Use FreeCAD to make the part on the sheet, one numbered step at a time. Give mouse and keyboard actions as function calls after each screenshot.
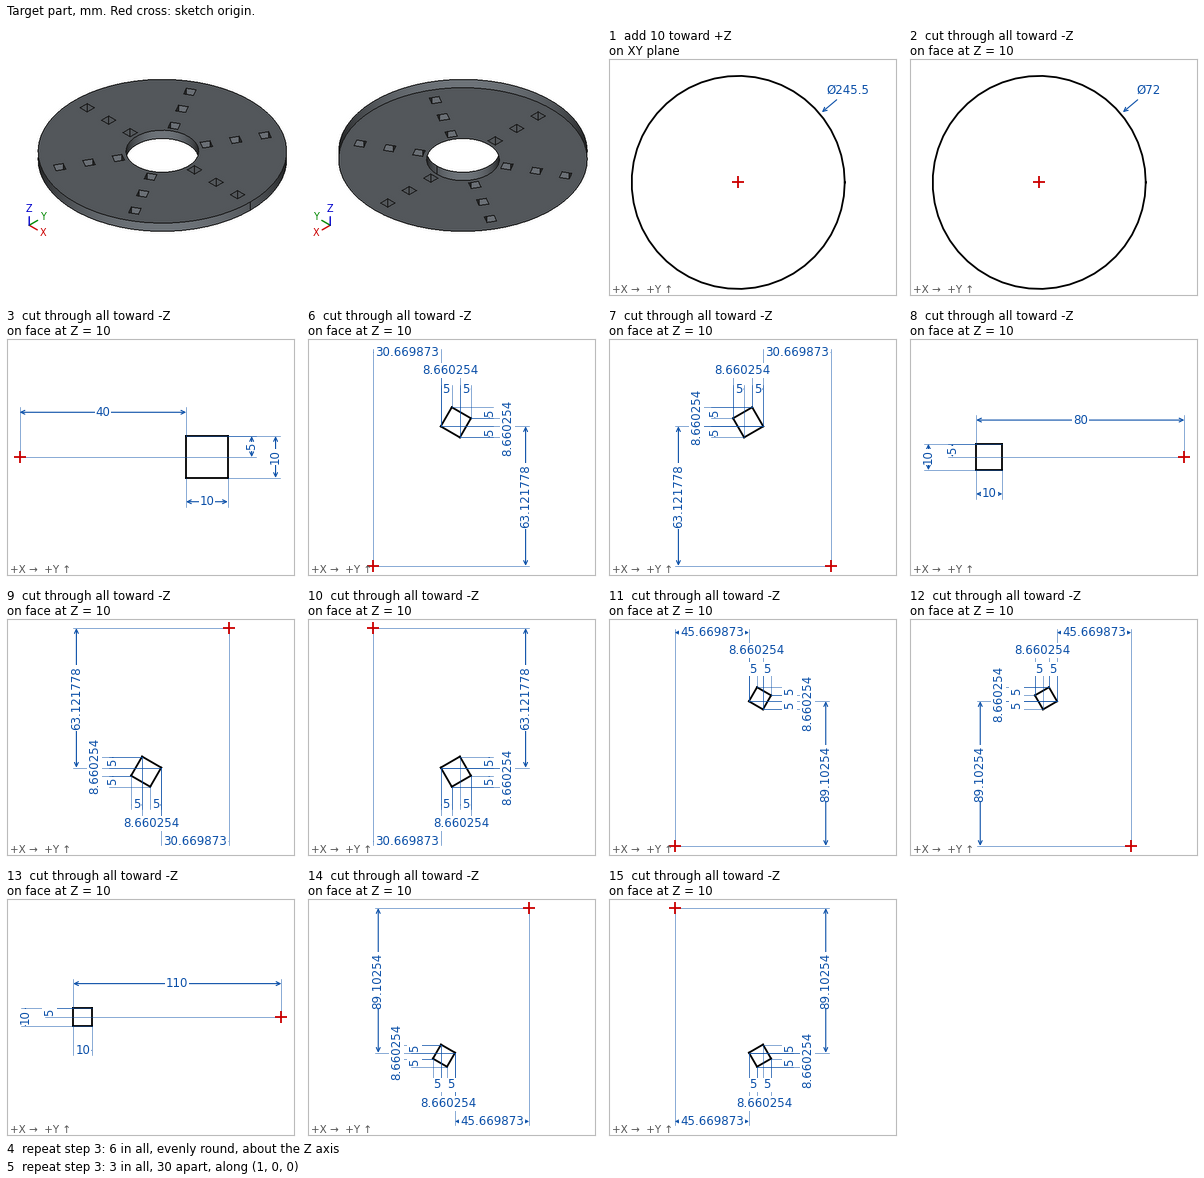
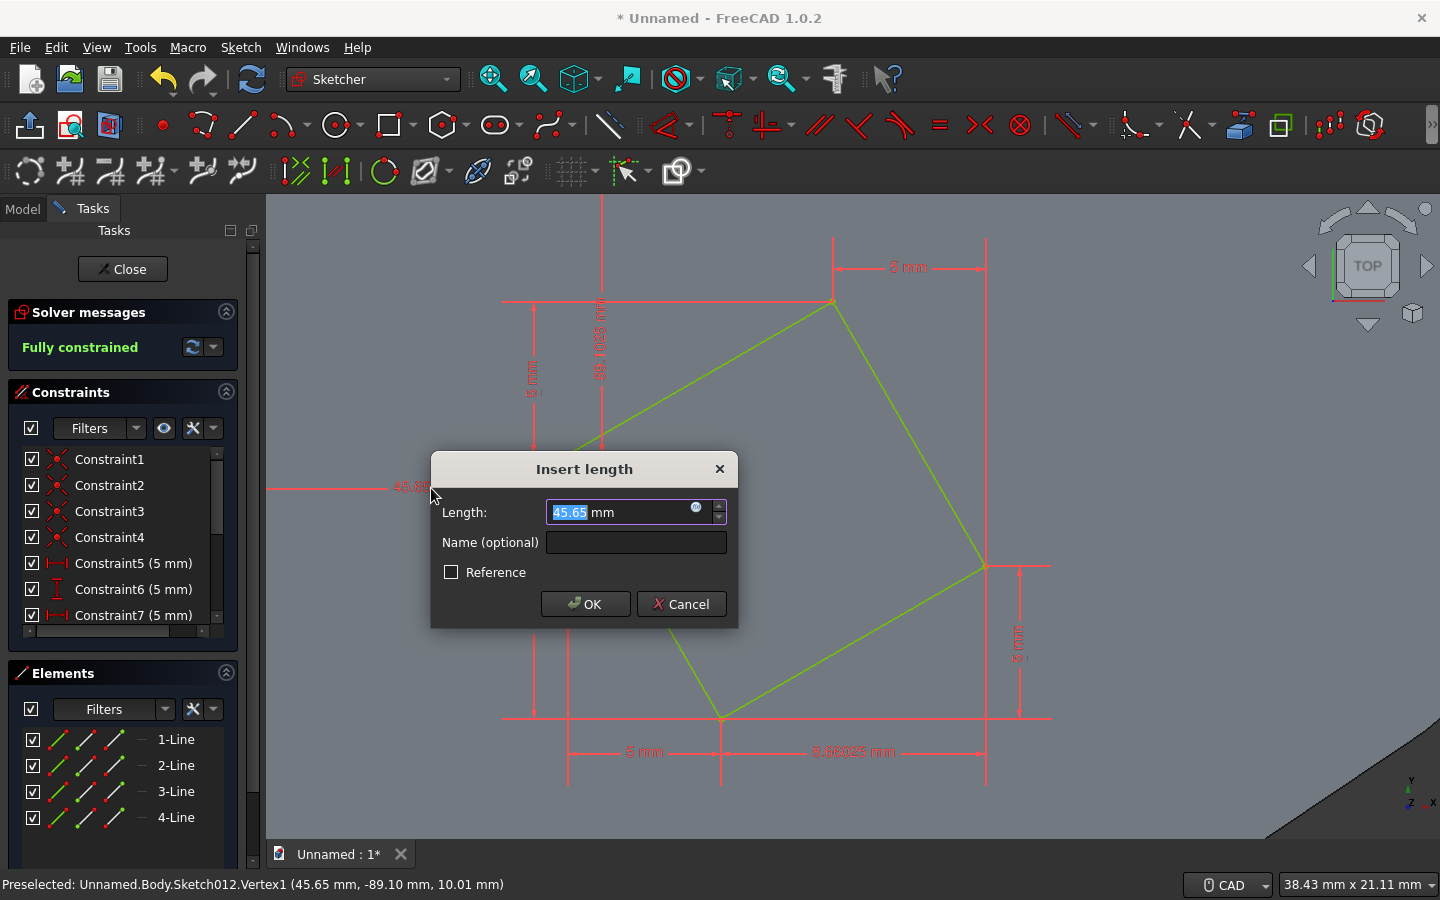
text(45.669873)
key(Return)
key(Escape)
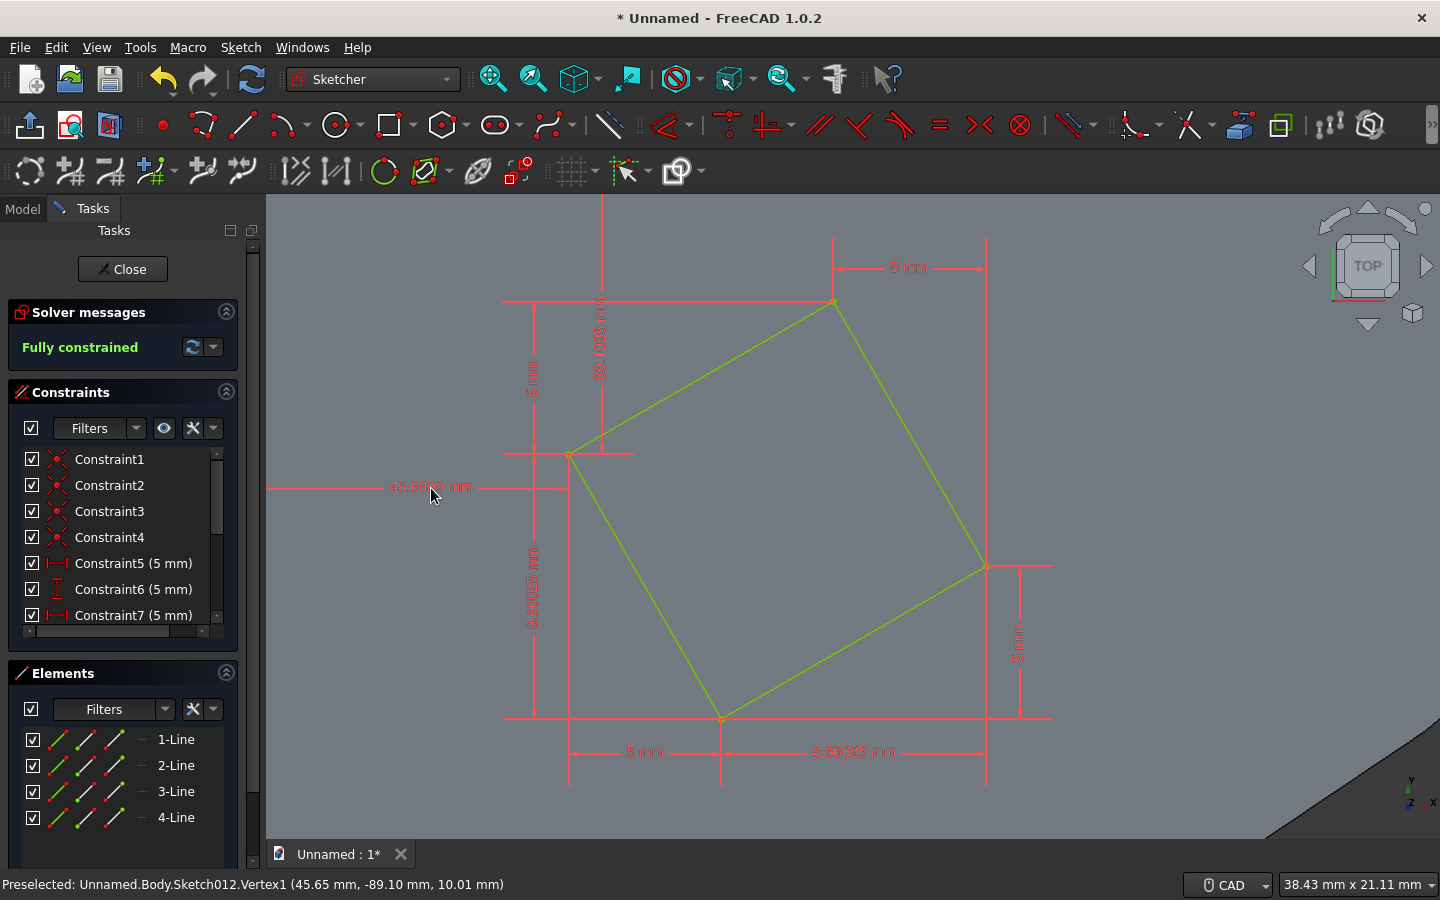
click(123, 269)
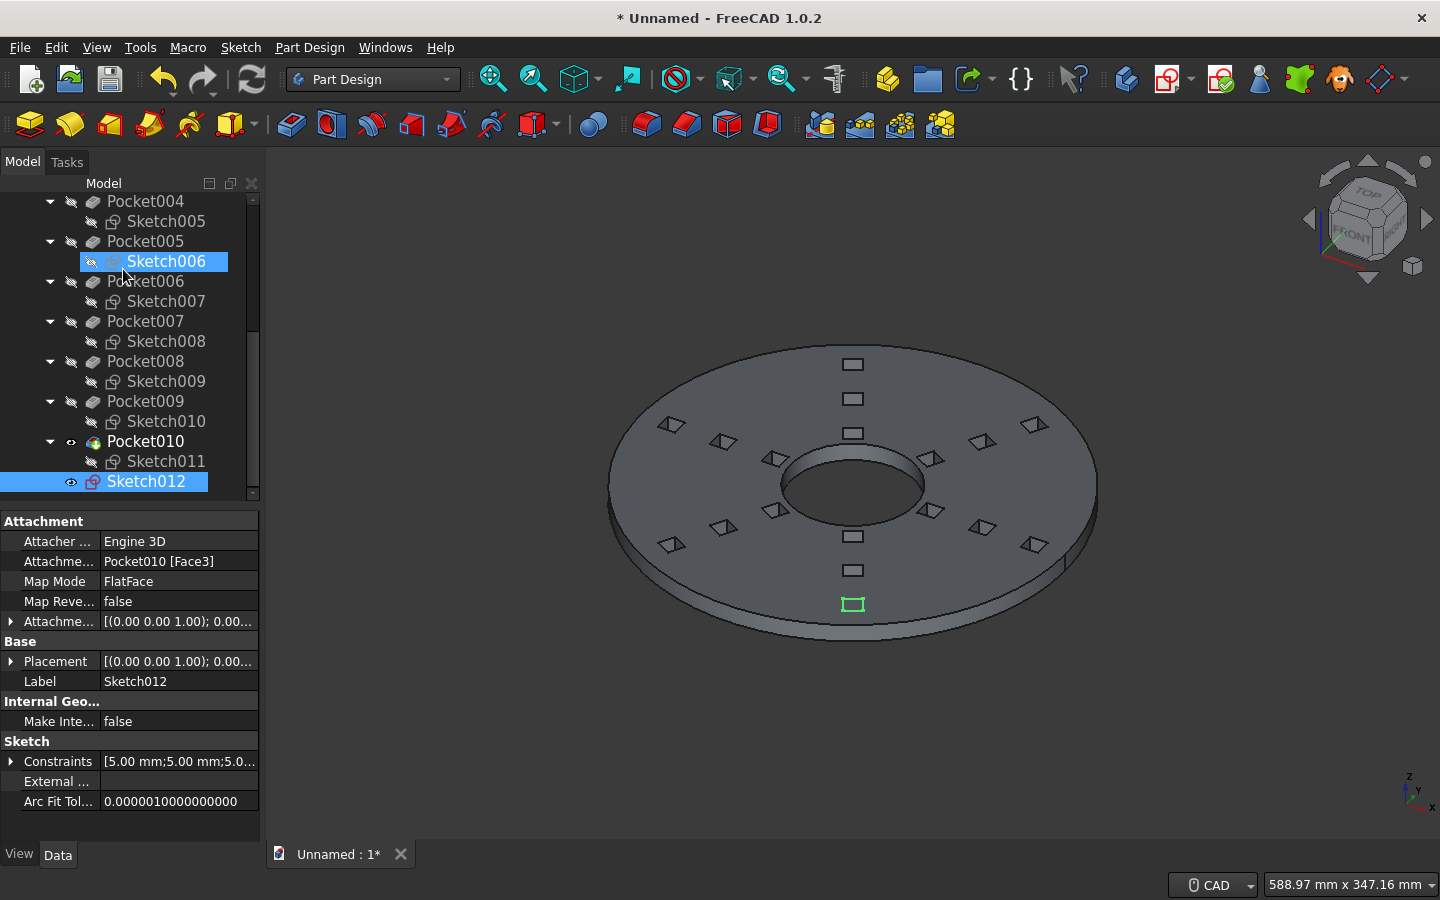
click(292, 124)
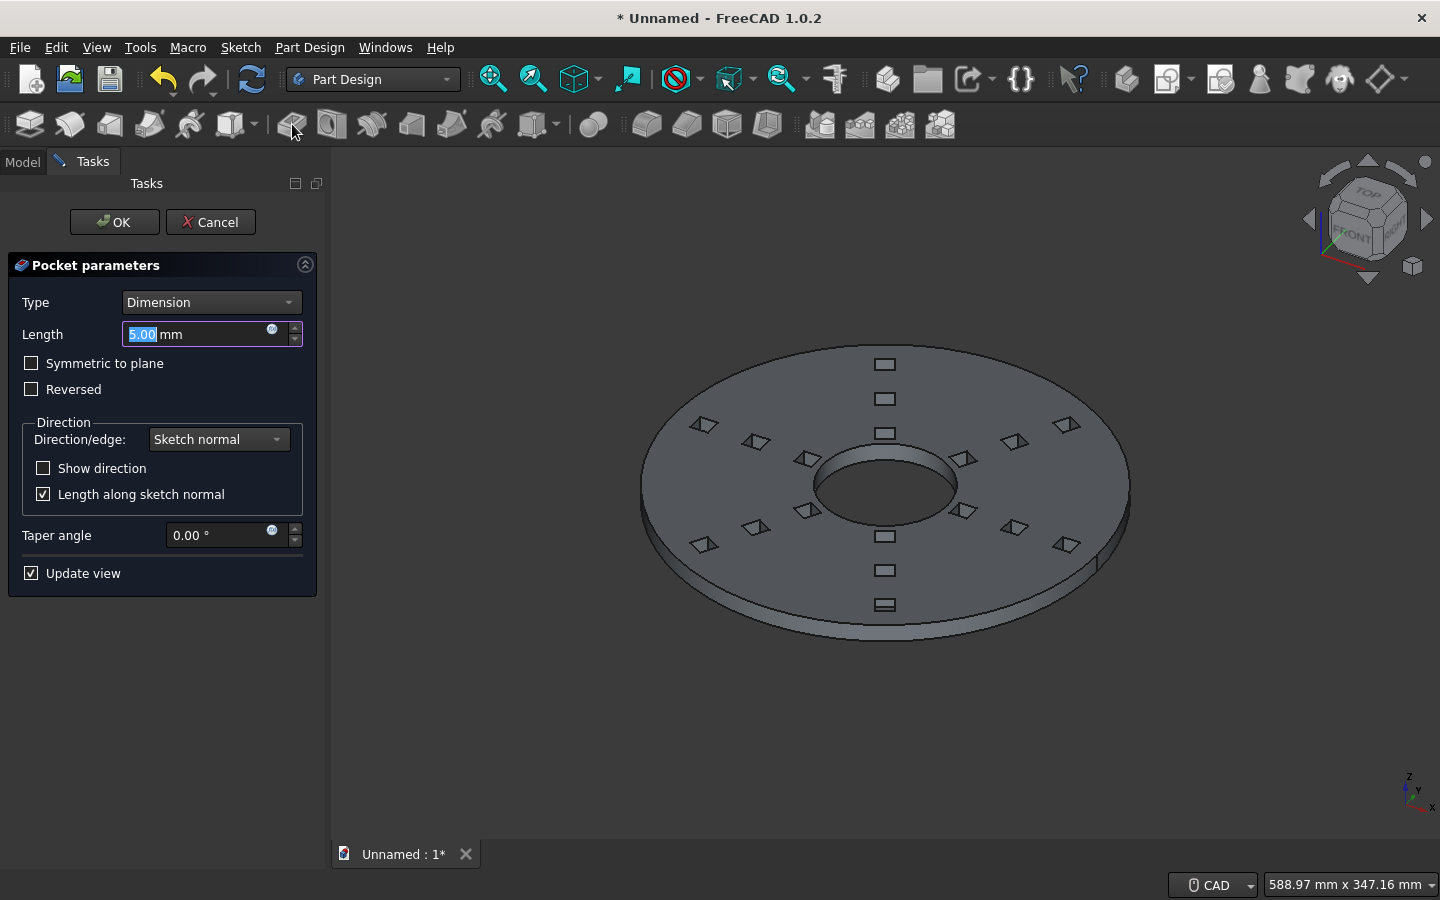
click(212, 302)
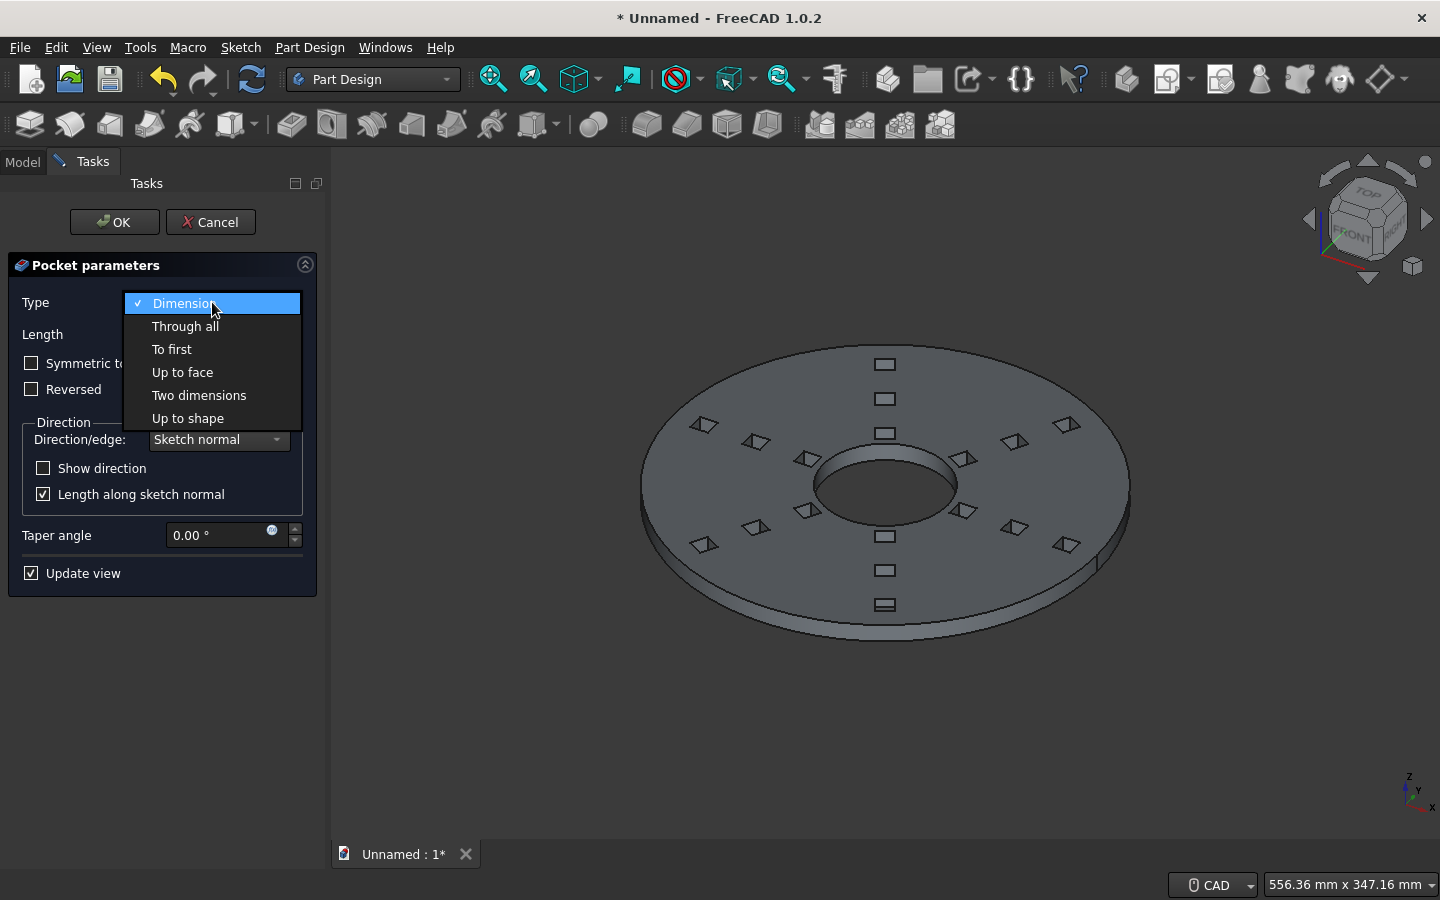
click(212, 326)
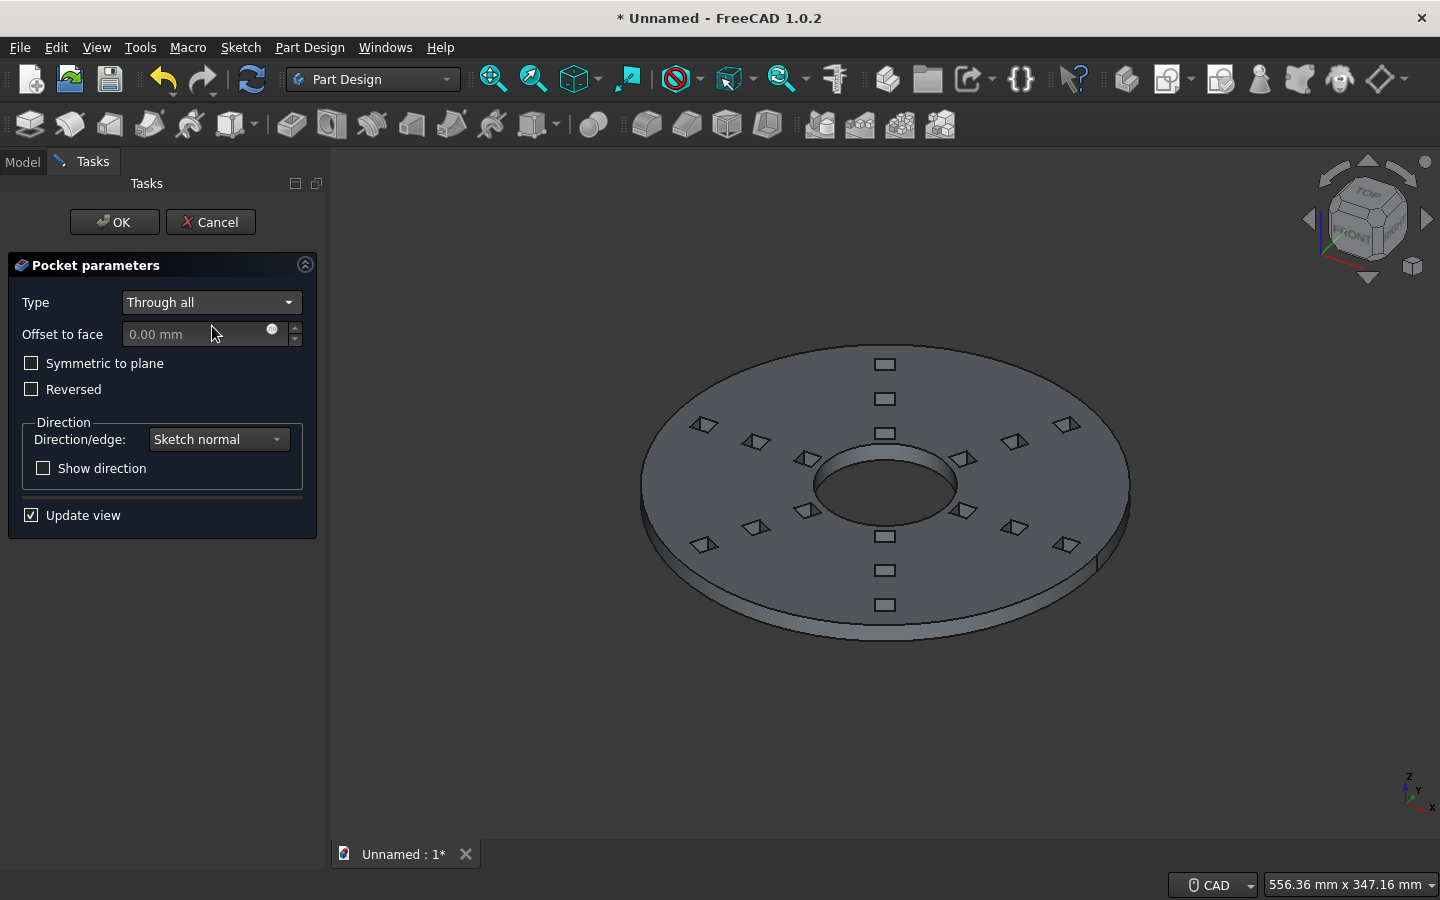
click(115, 222)